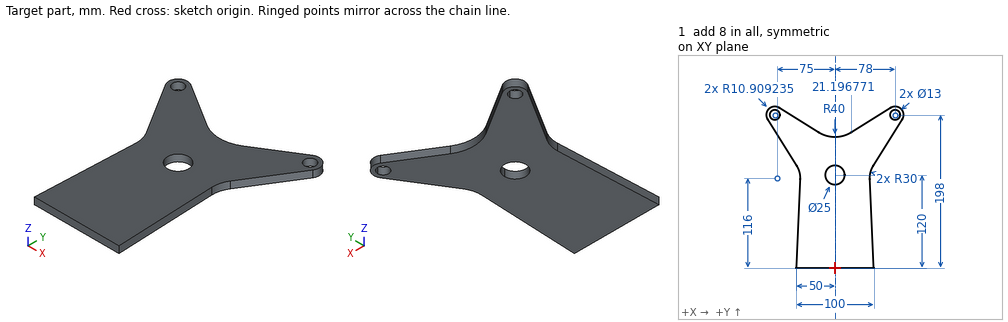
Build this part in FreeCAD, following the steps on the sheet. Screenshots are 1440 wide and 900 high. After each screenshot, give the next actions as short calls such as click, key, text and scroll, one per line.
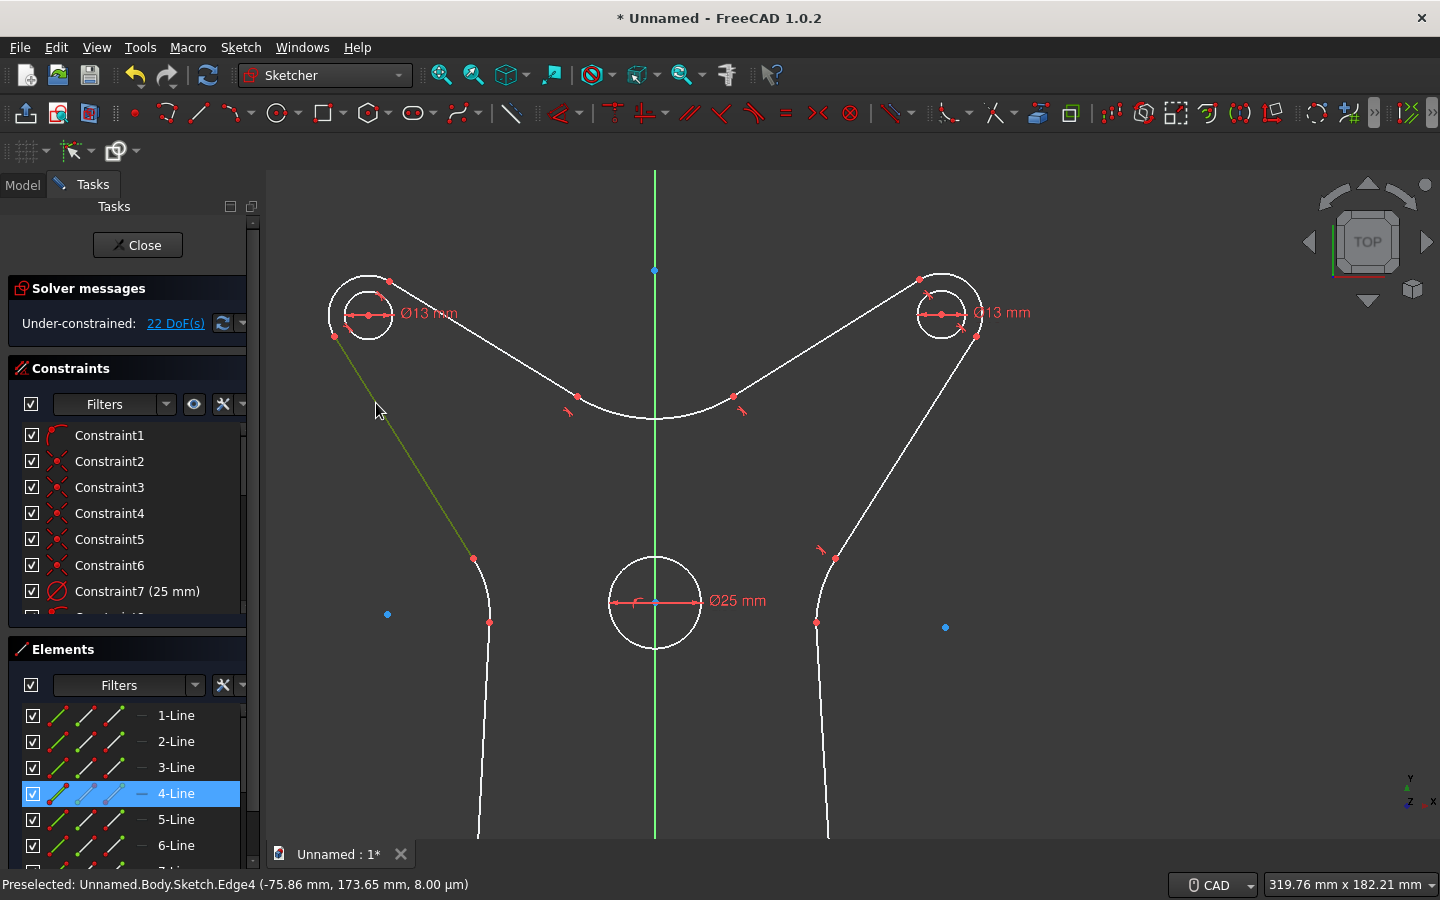
click(489, 603)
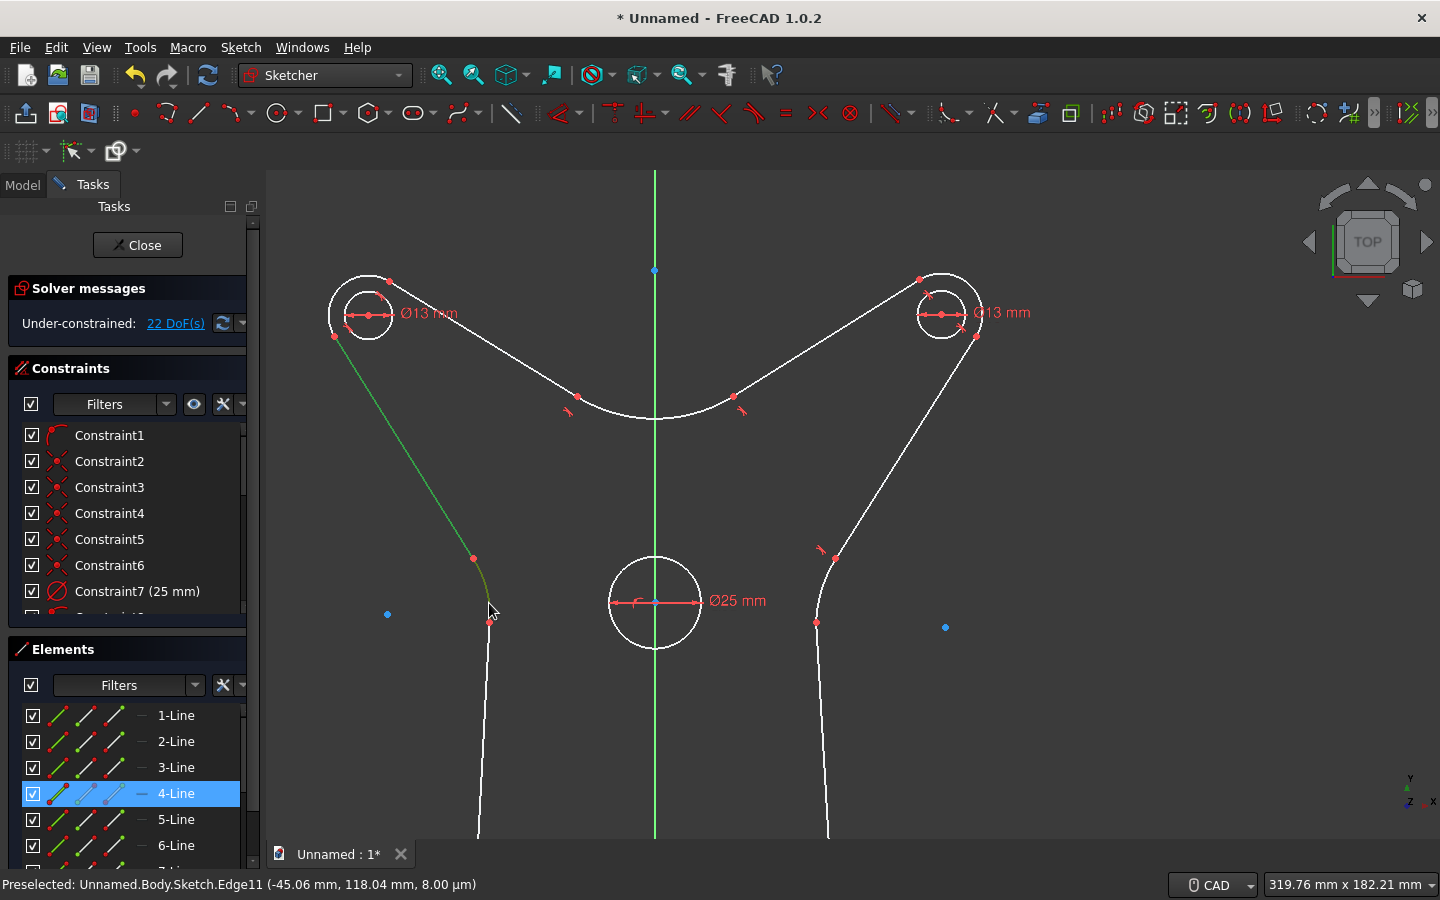
click(754, 114)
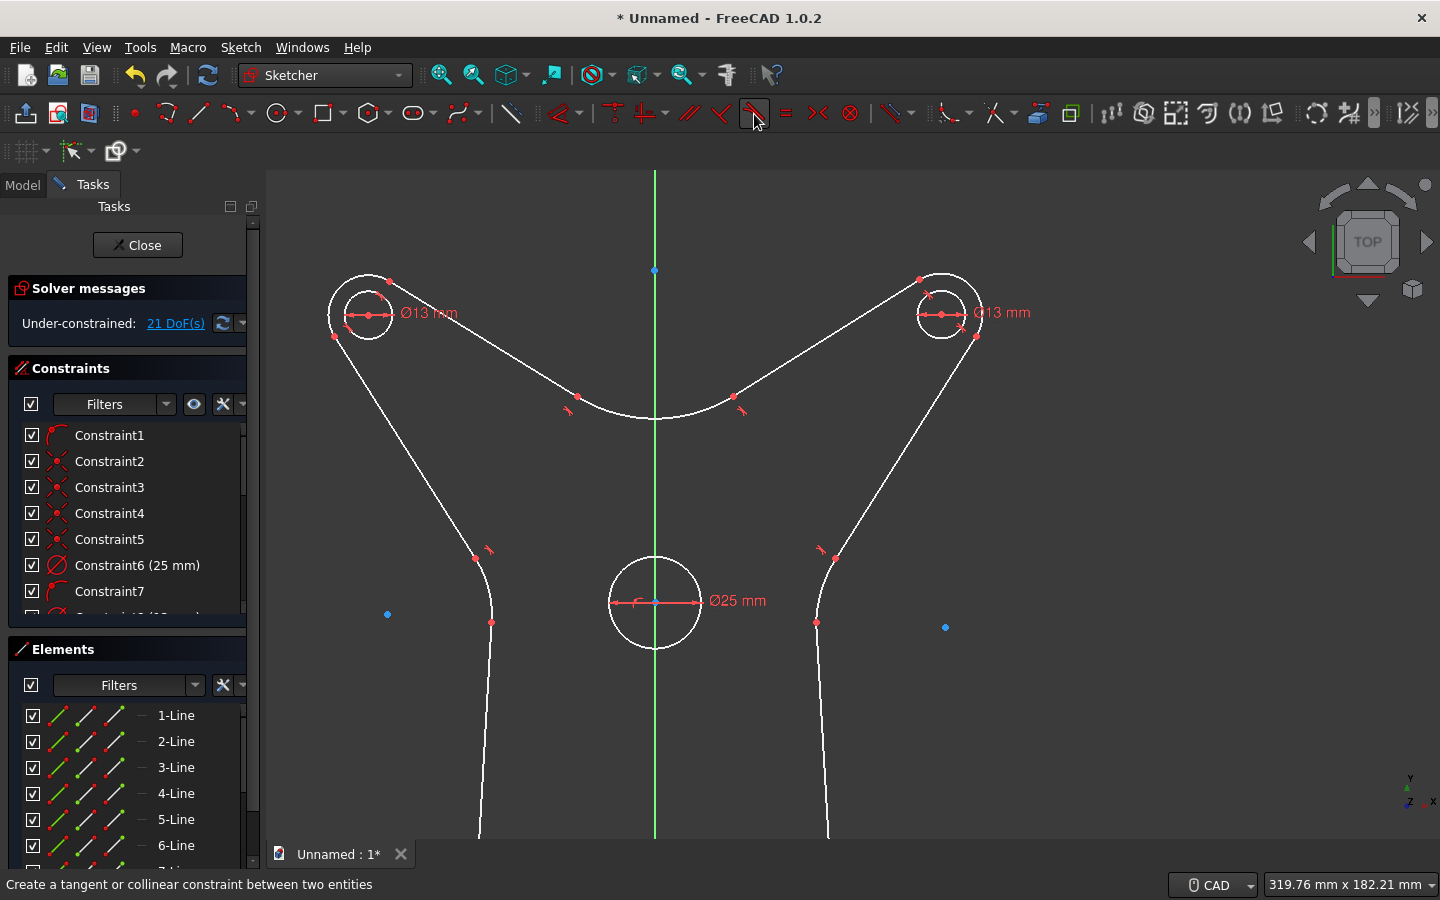
click(484, 748)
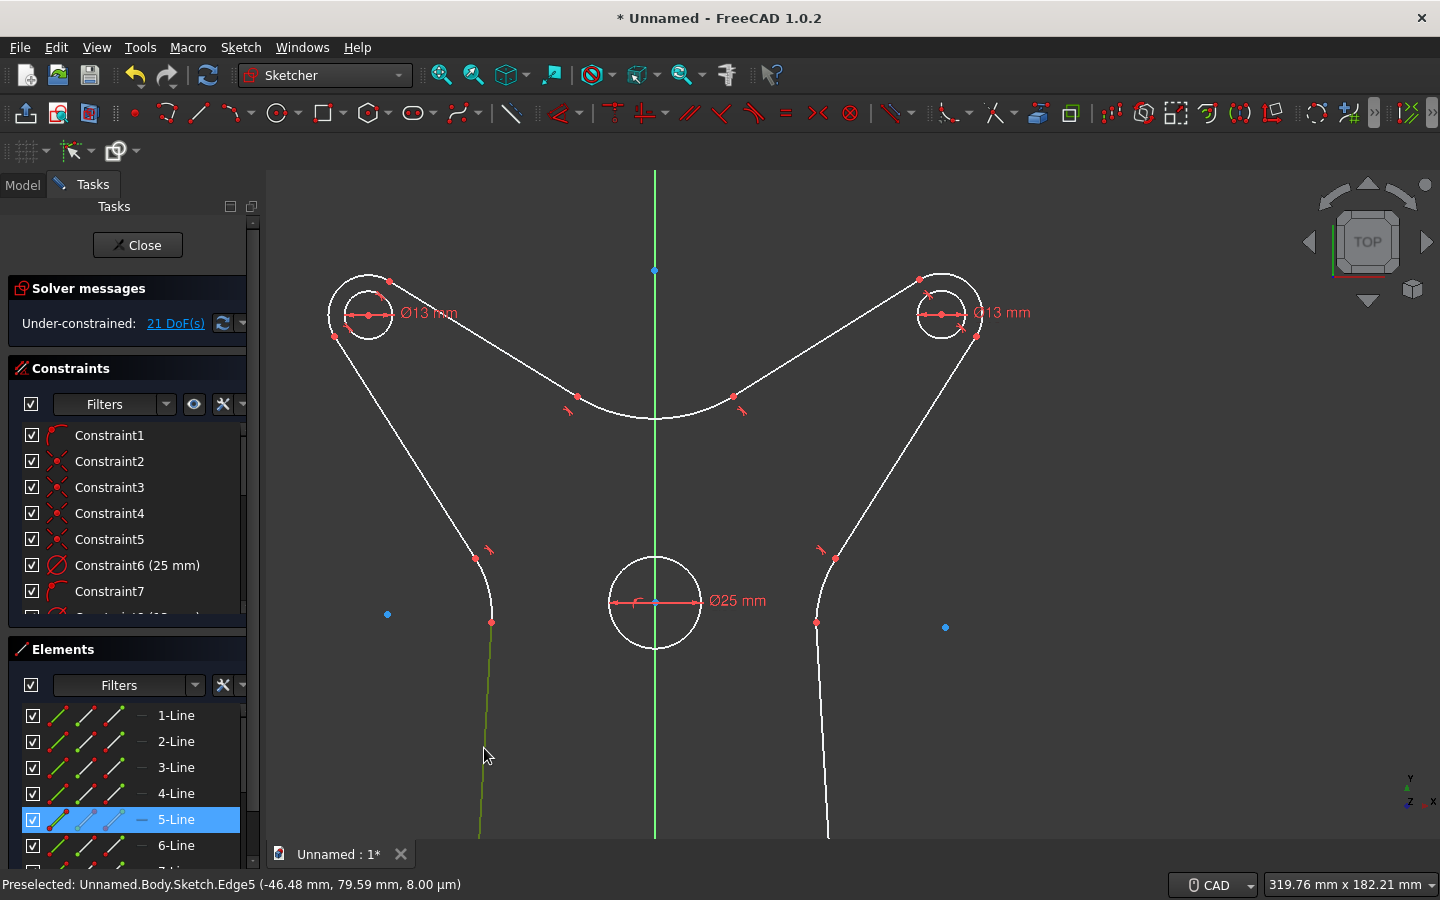
click(491, 603)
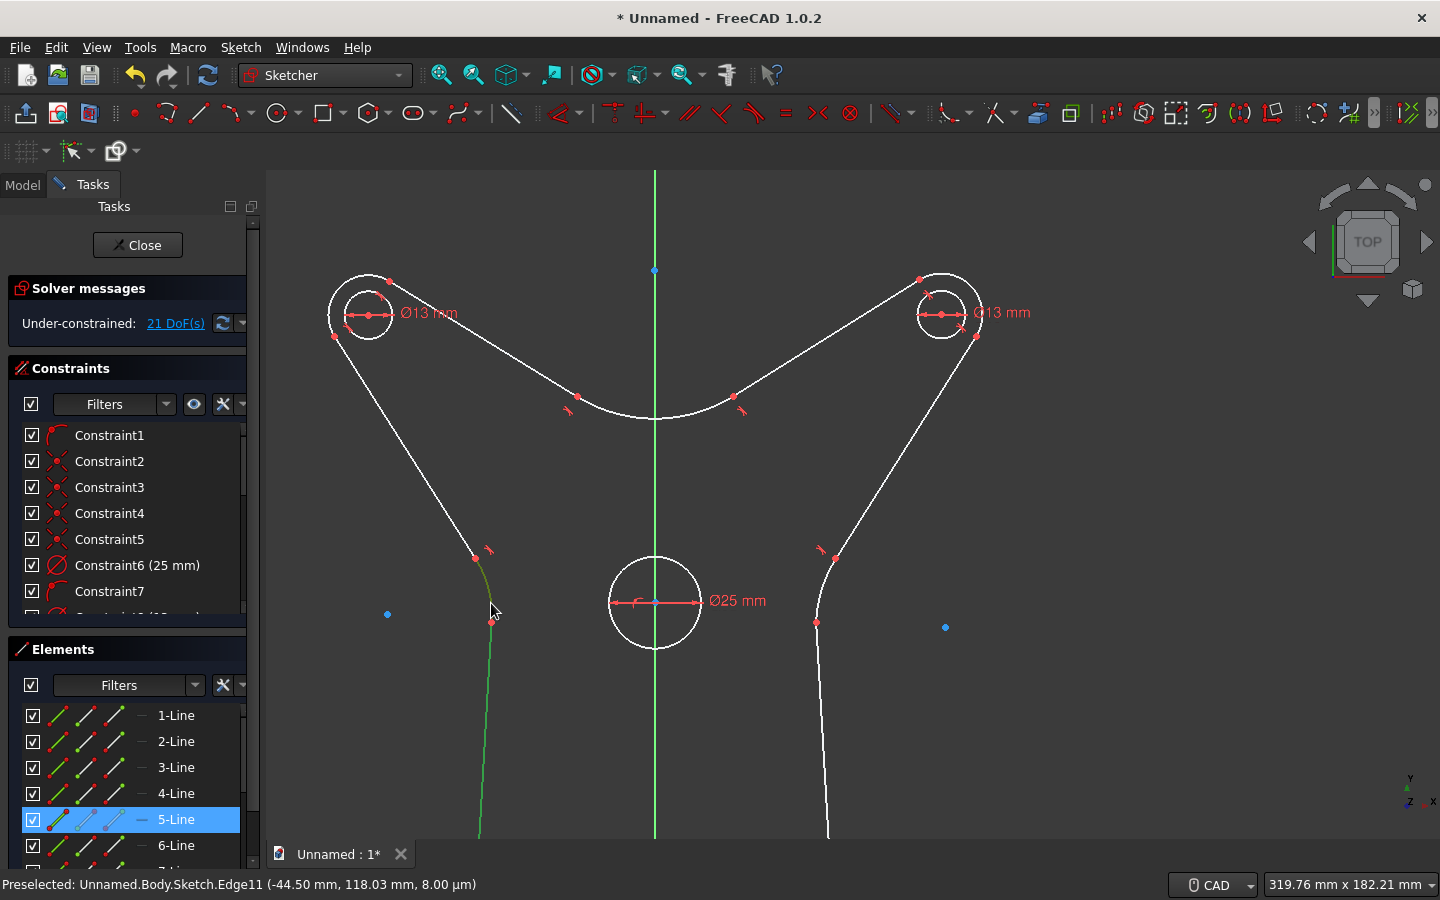
click(754, 114)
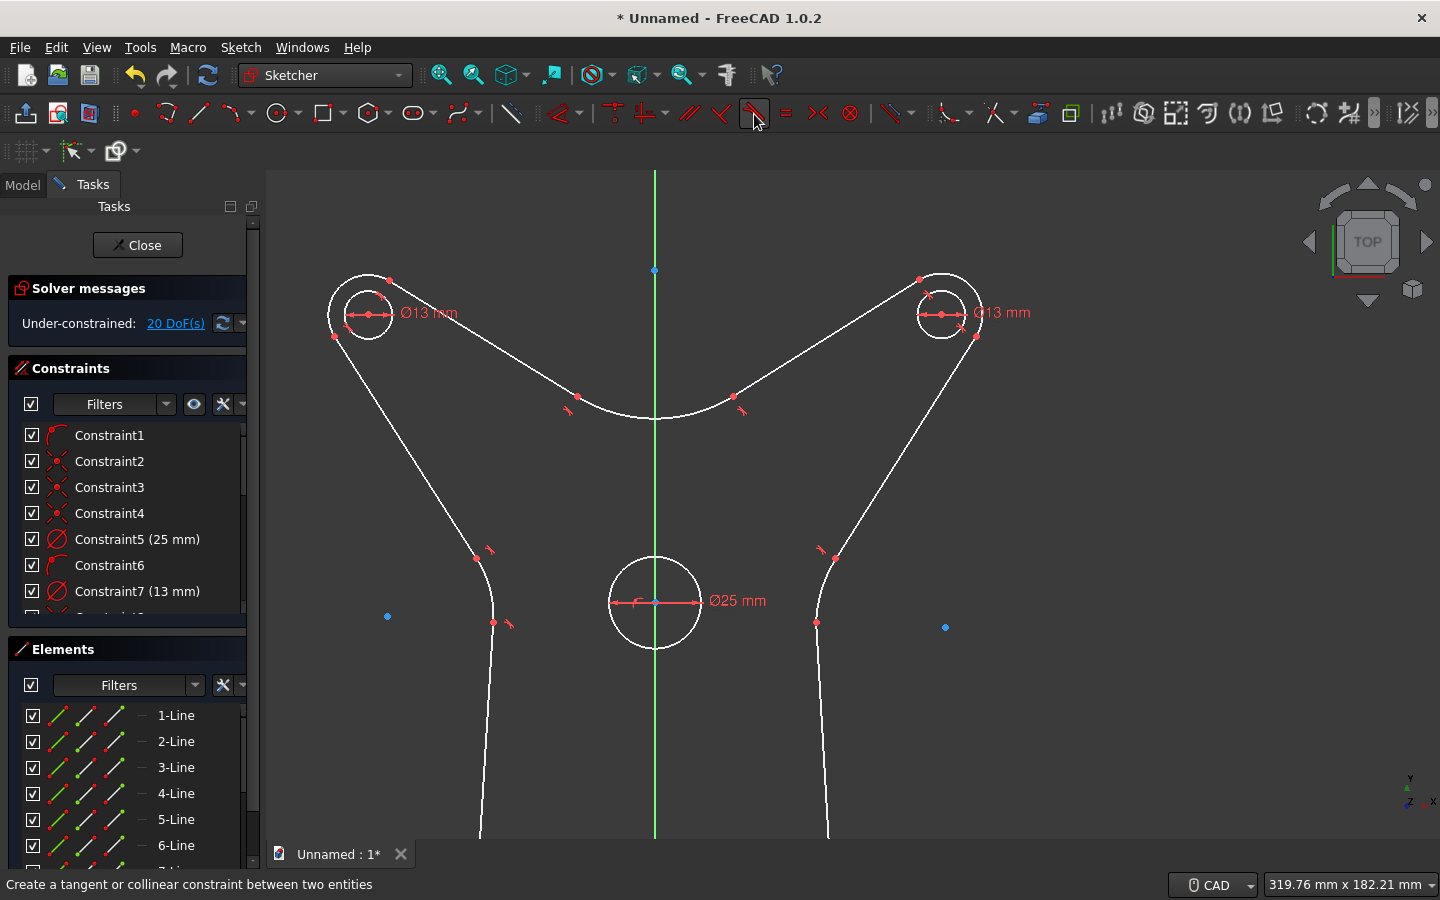
click(823, 744)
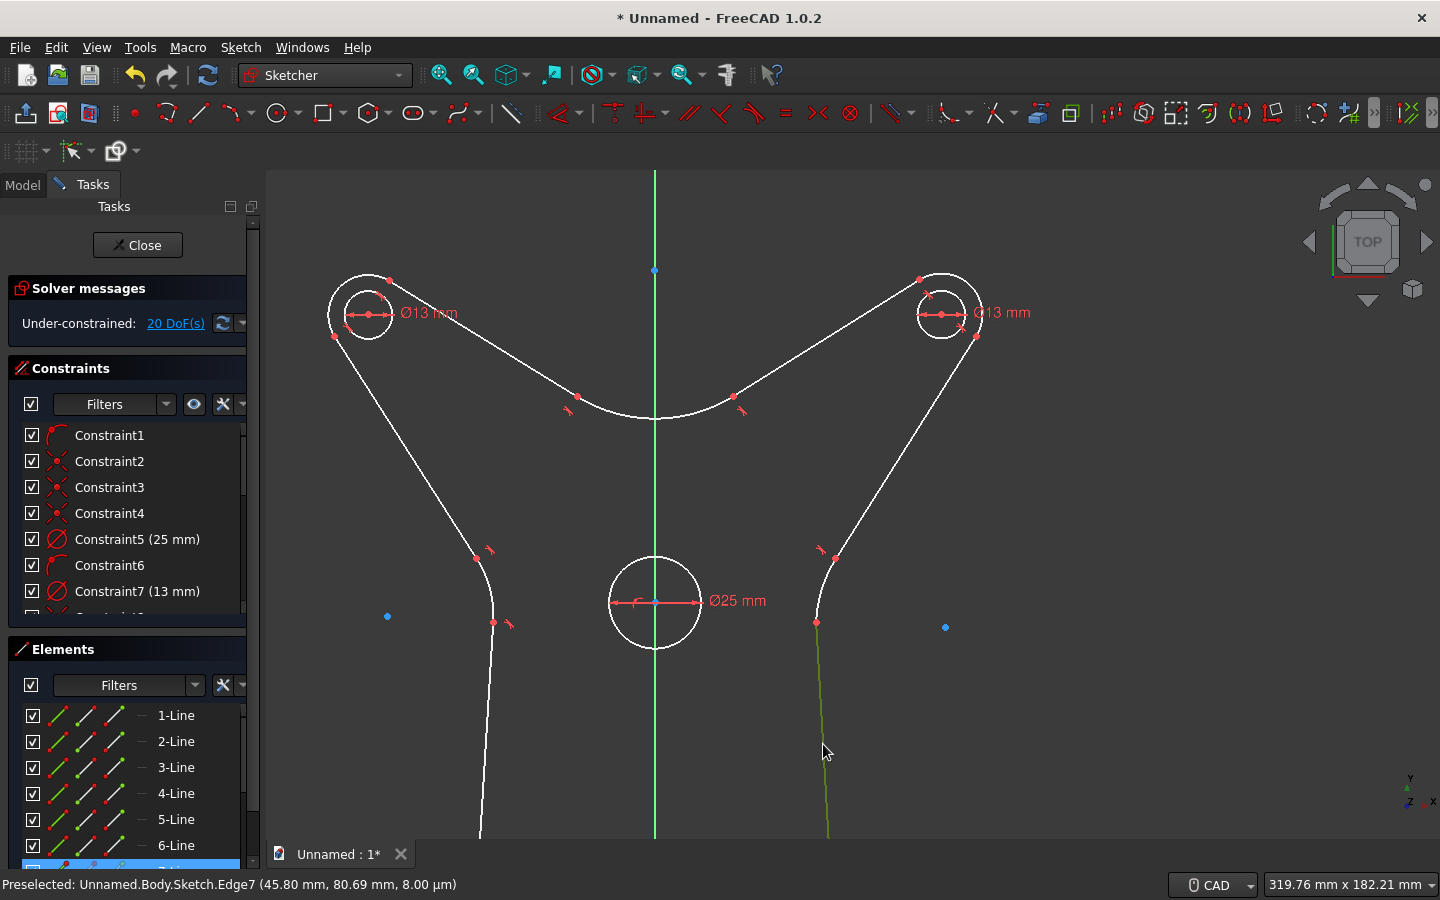
click(826, 577)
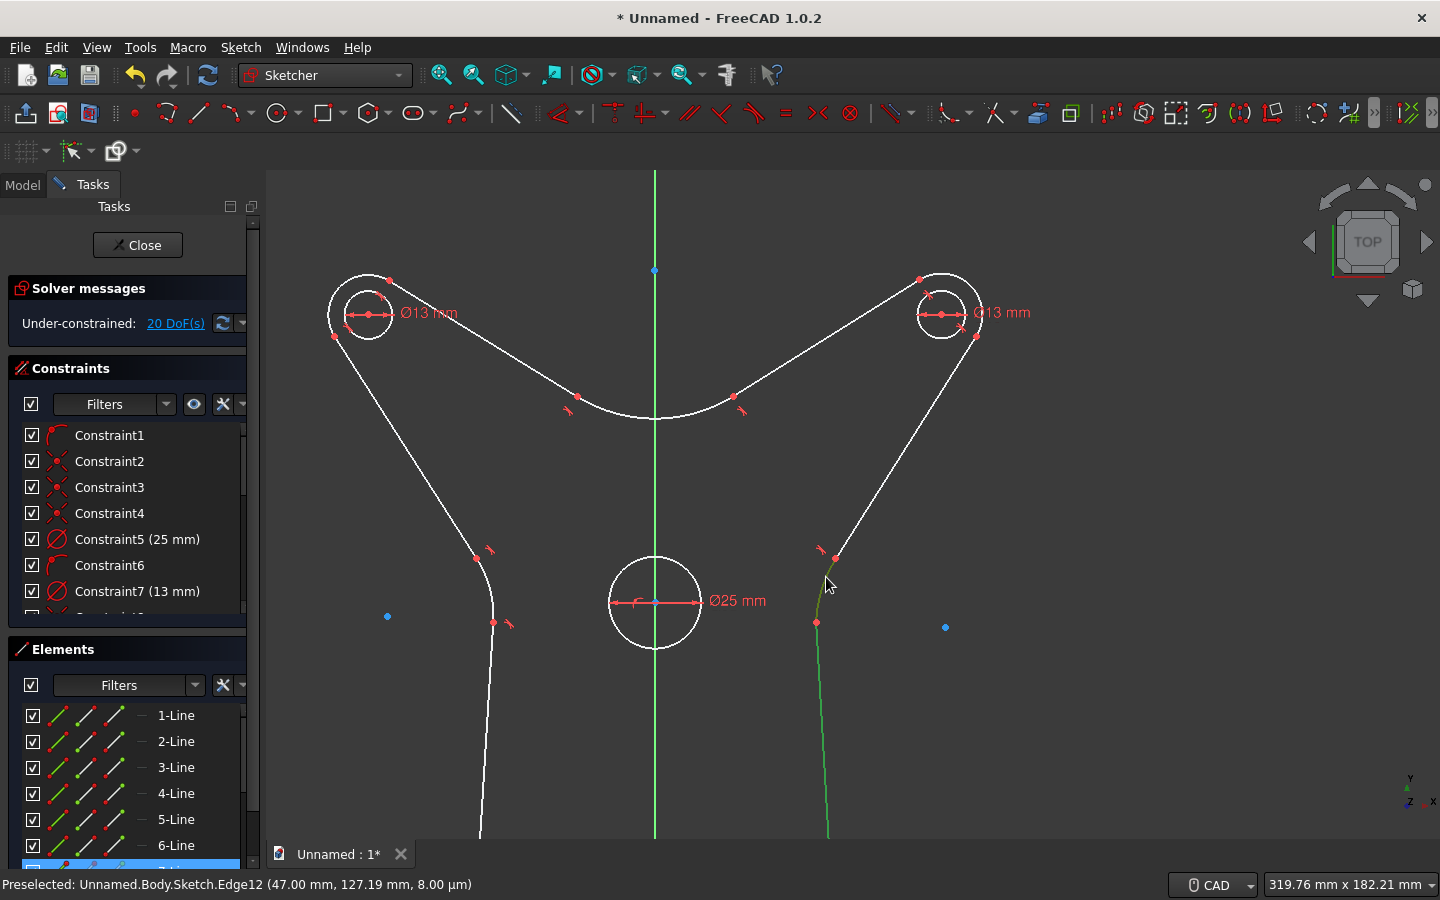
click(754, 114)